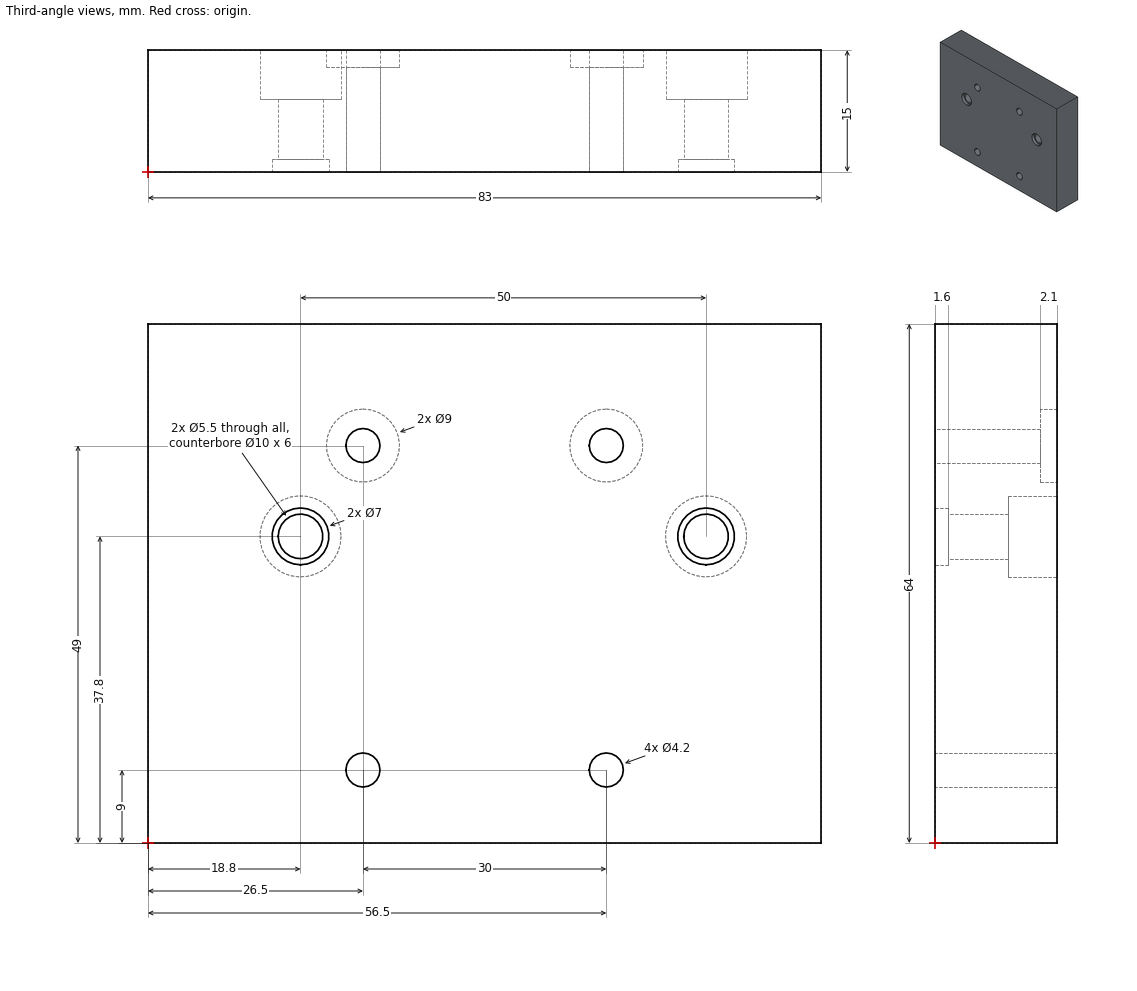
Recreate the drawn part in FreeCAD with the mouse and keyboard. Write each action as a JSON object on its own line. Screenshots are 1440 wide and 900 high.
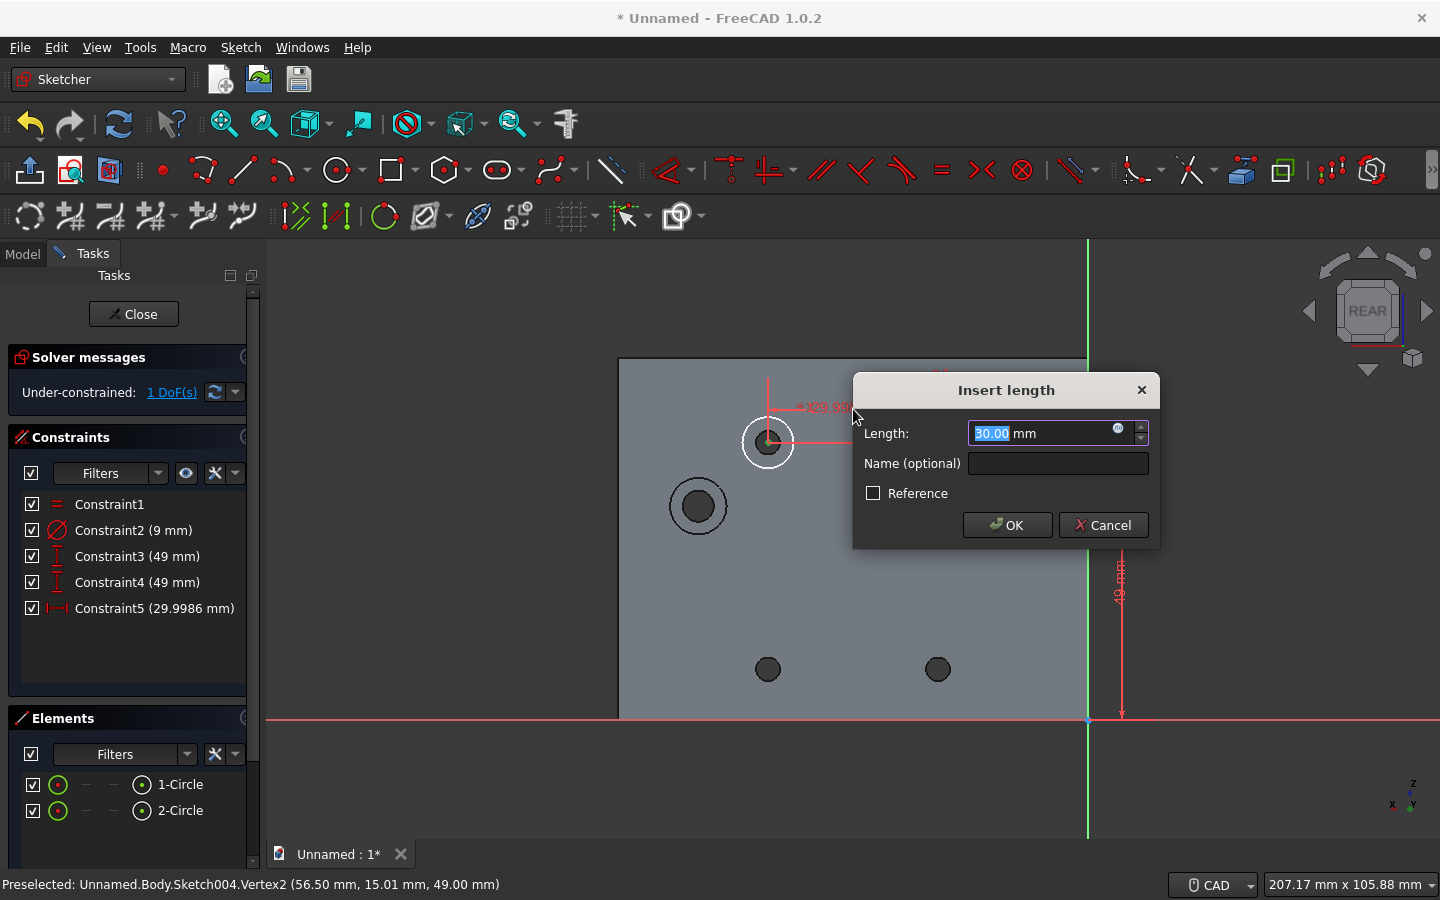
{"action": "type", "text": "30"}
{"action": "key", "text": "Return"}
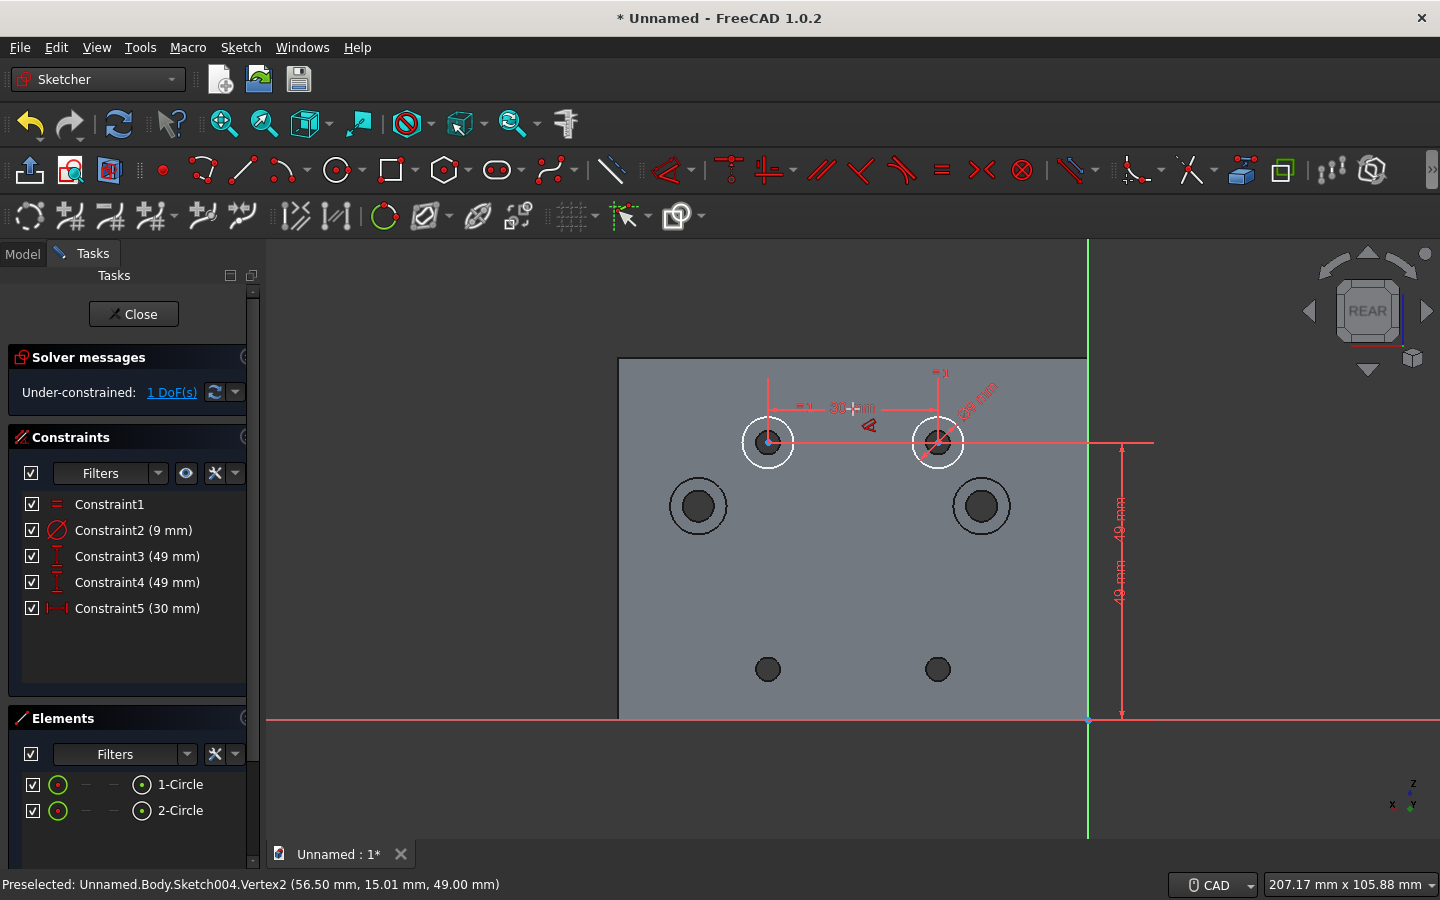
{"action": "left_click", "coordinate": [938, 443]}
{"action": "left_click", "coordinate": [1013, 754]}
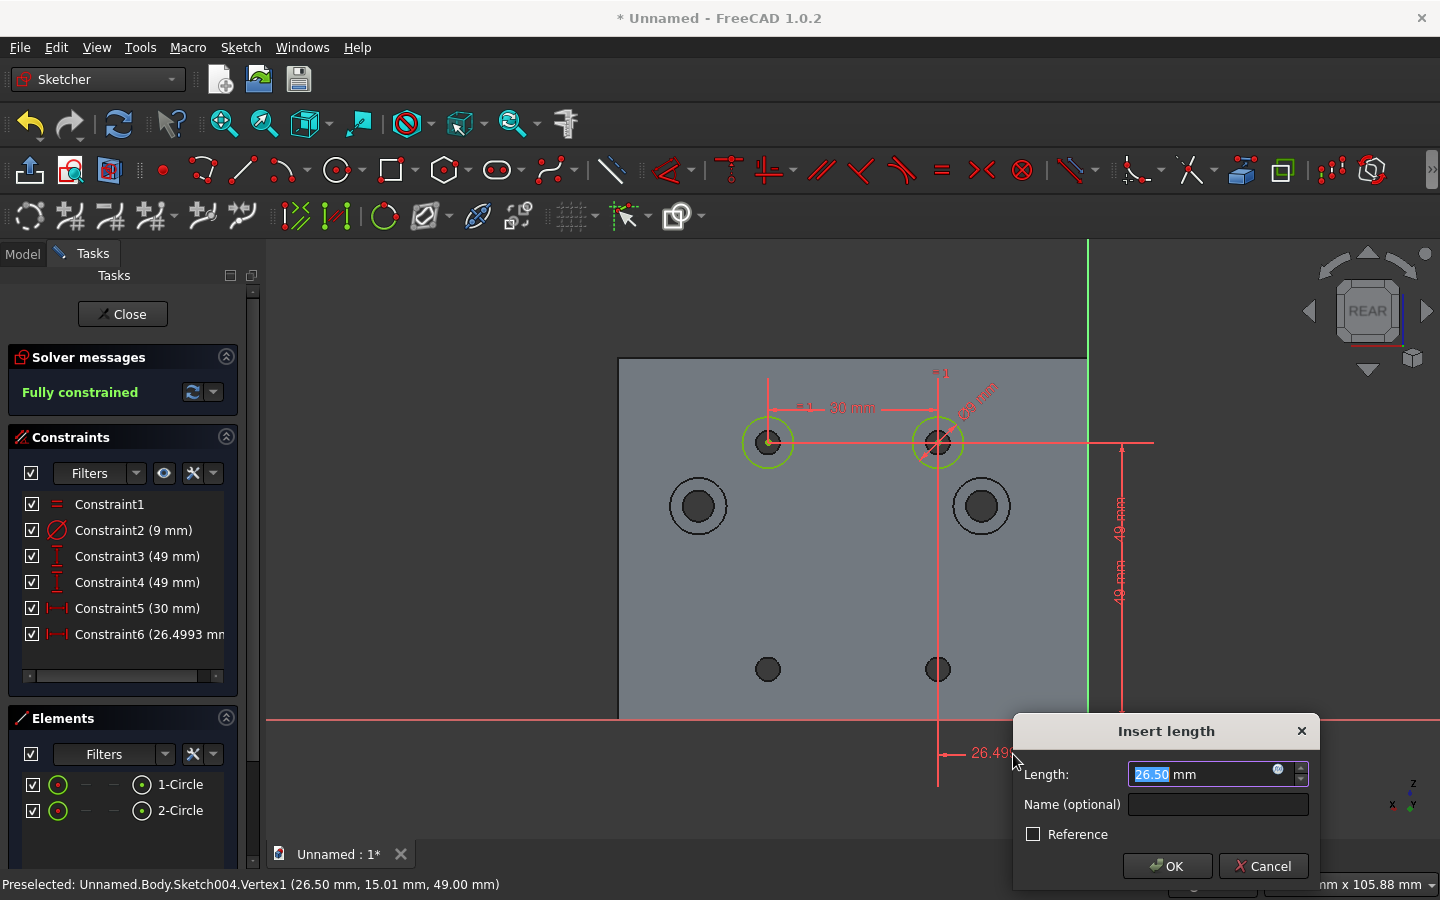
{"action": "type", "text": "26.5"}
{"action": "key", "text": "Return"}
{"action": "key", "text": "Escape"}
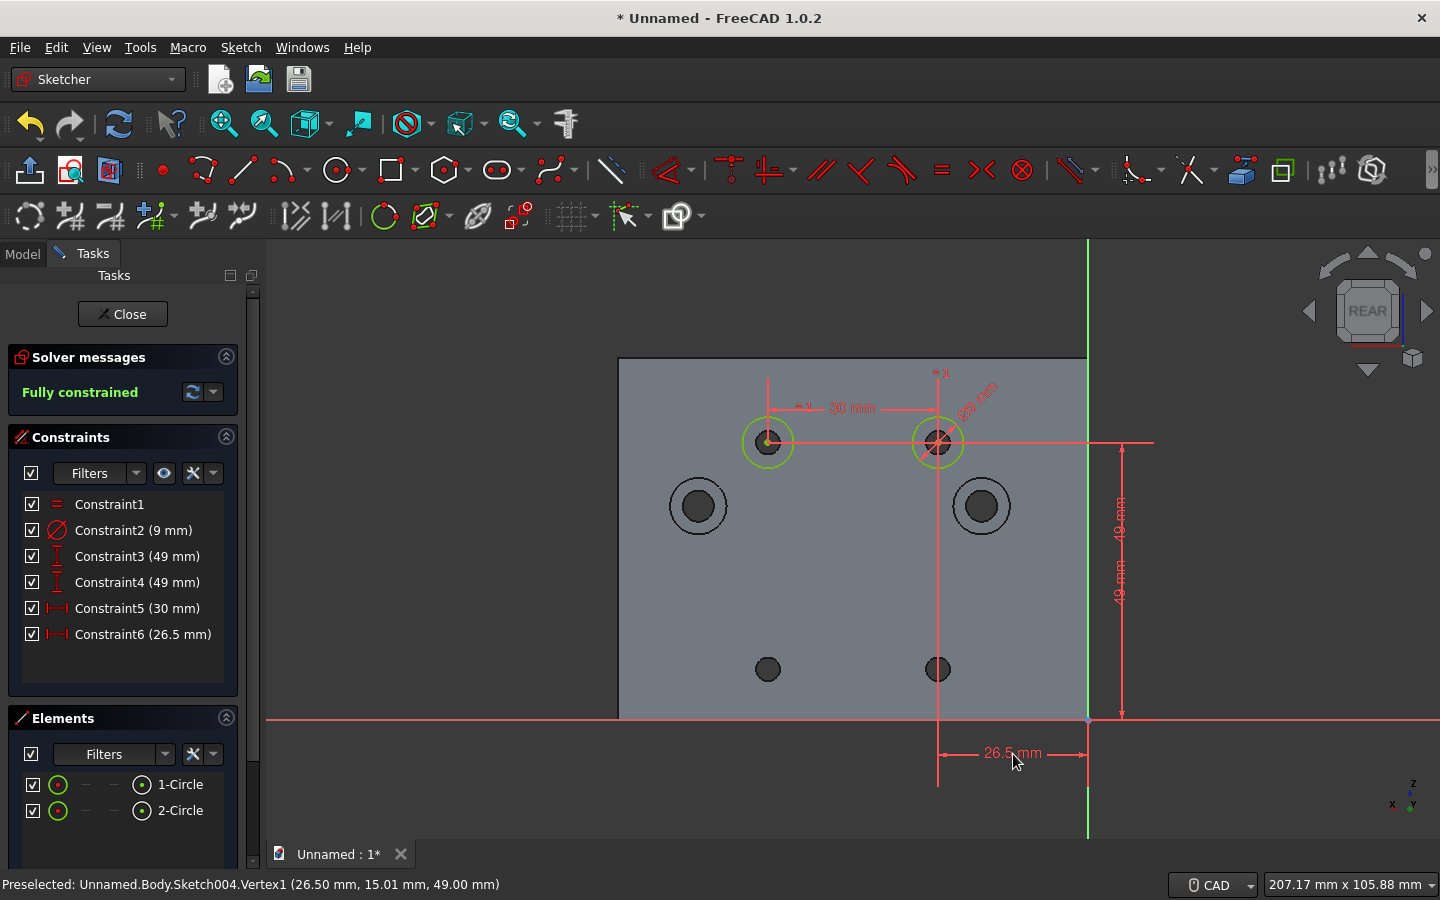
{"action": "left_click", "coordinate": [123, 314]}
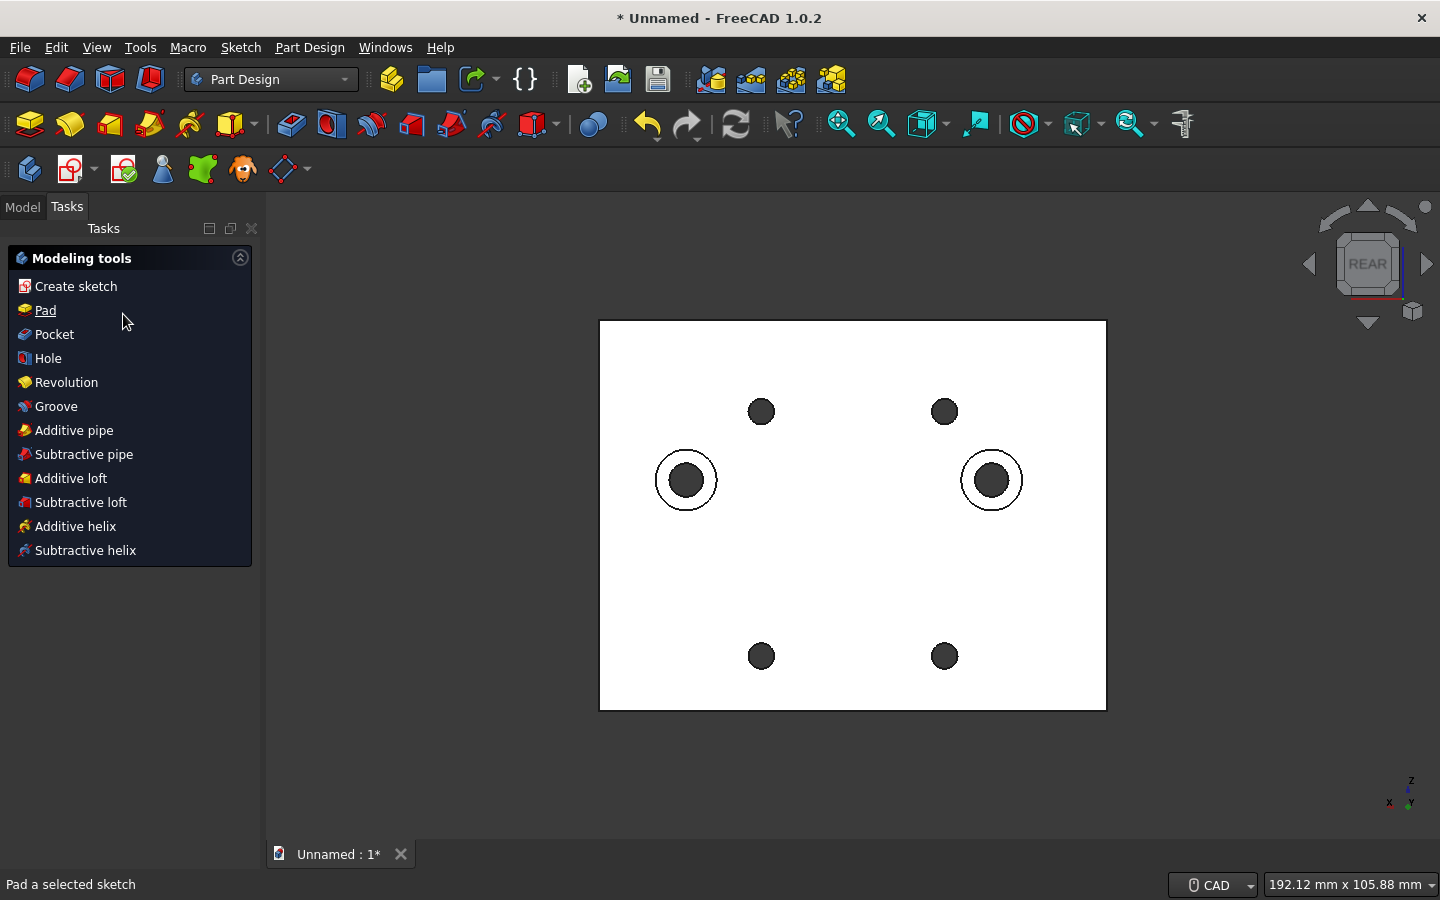
{"action": "left_click", "coordinate": [292, 124]}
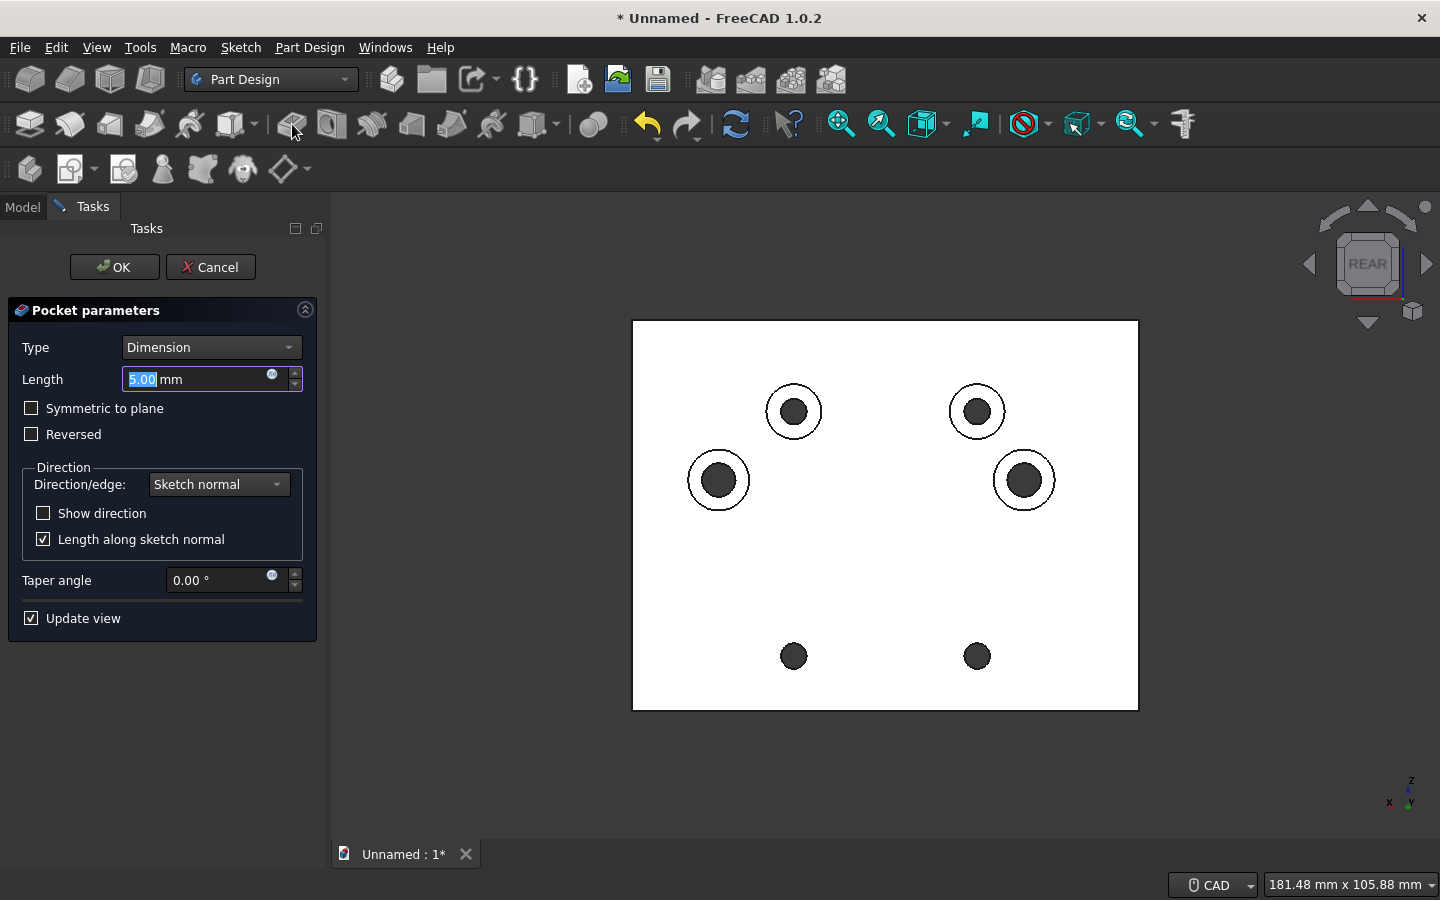
{"action": "type", "text": "2.1"}
{"action": "key", "text": "Tab"}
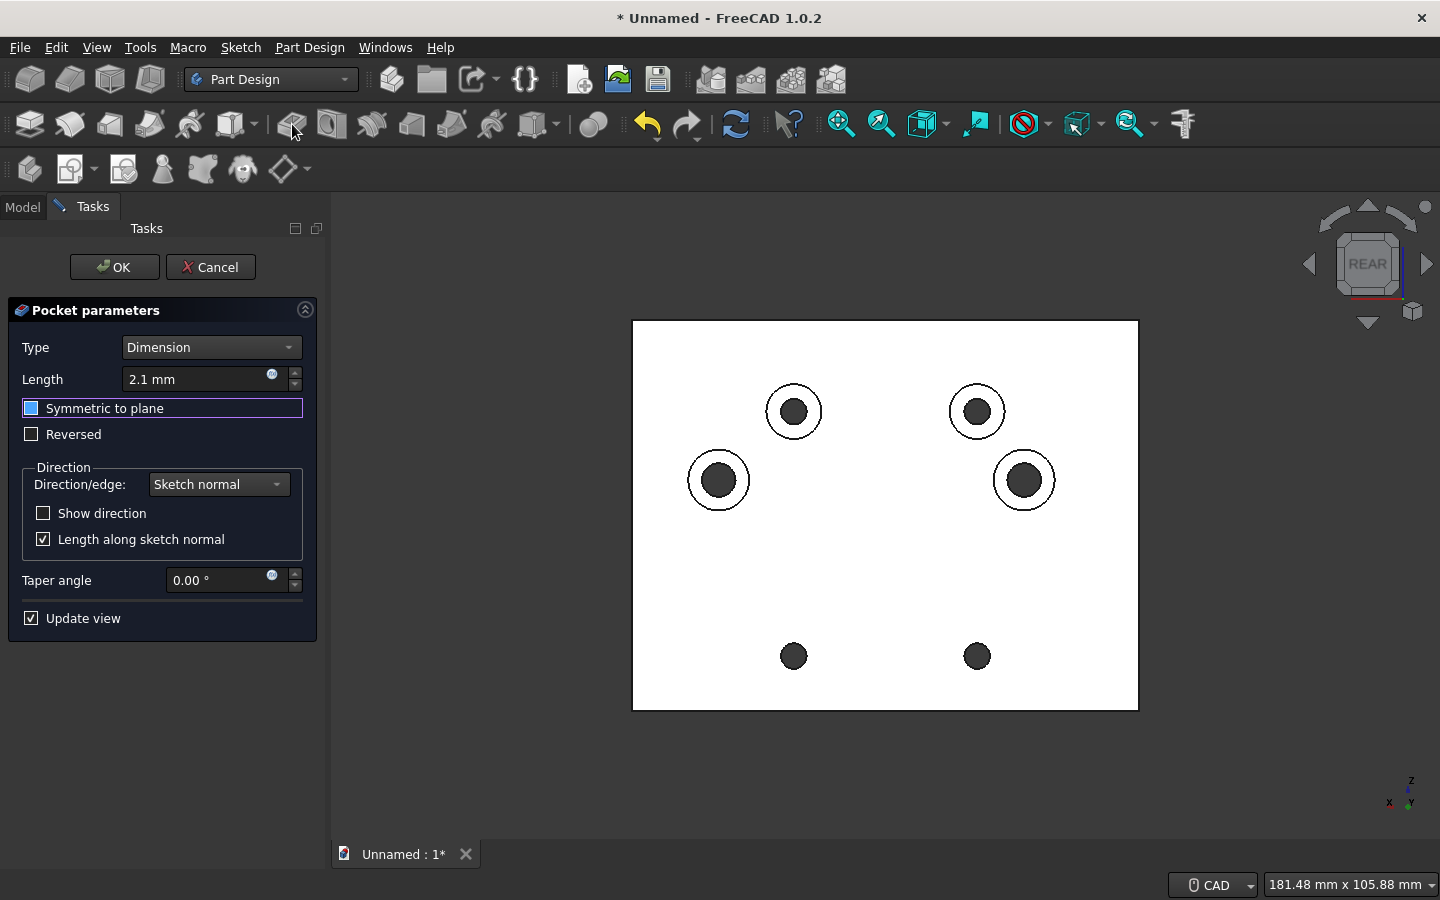
{"action": "left_click", "coordinate": [115, 267]}